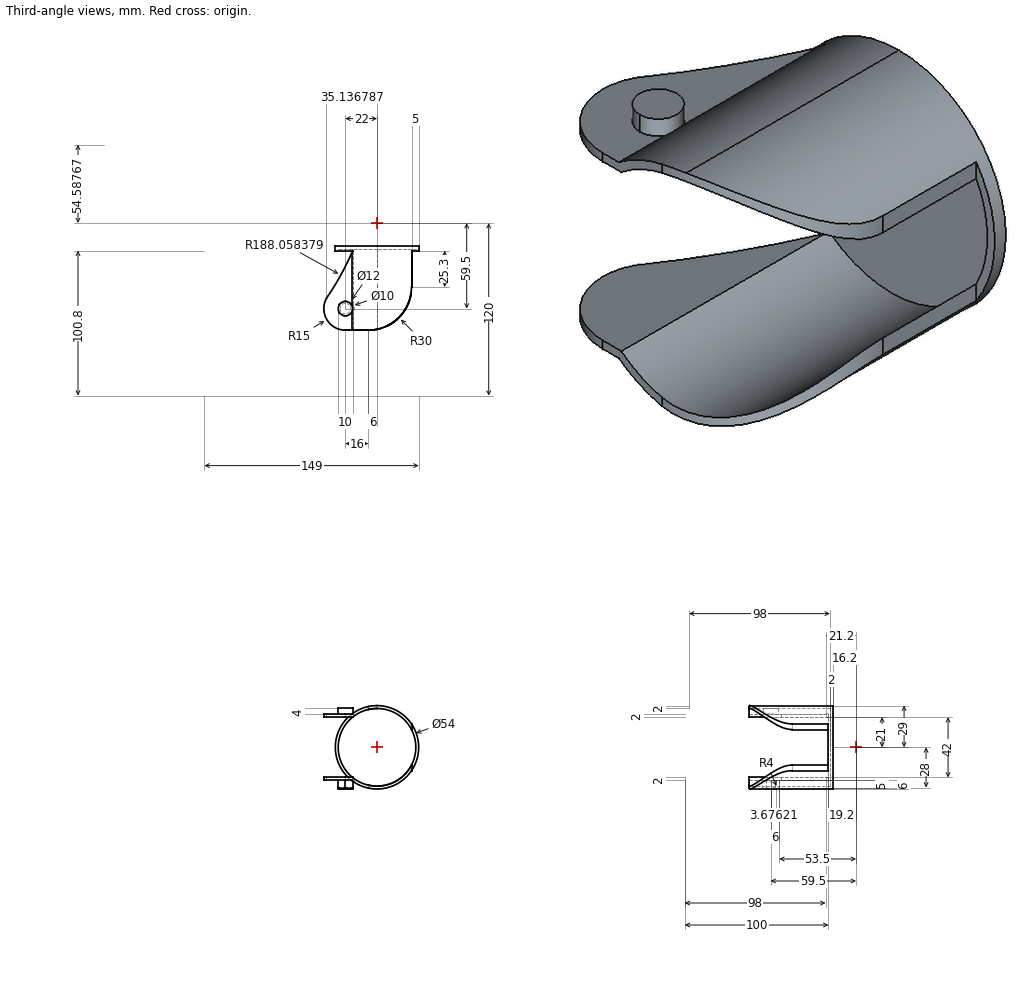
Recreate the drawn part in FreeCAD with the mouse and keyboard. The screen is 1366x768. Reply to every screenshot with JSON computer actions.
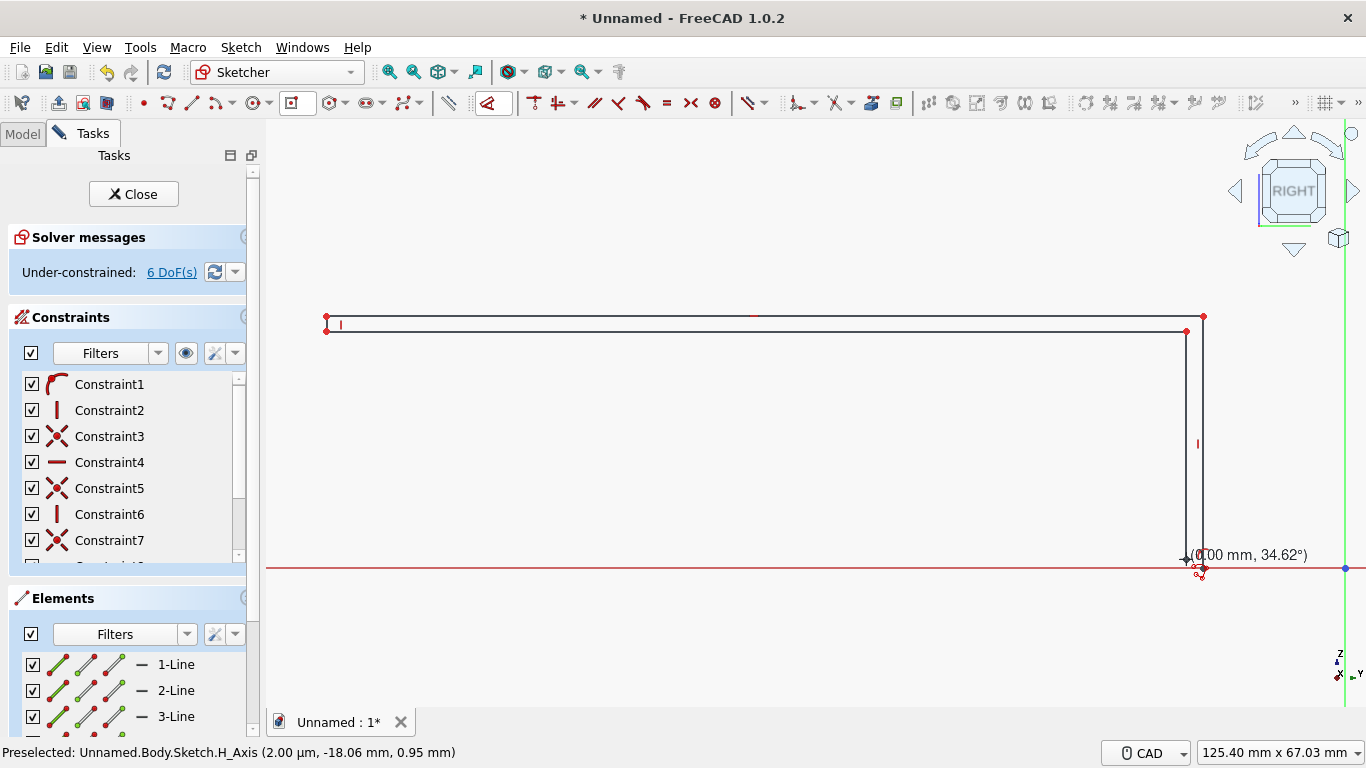
{"action": "scroll", "coordinate": [568, 356], "scroll_direction": "down", "scroll_amount": 2}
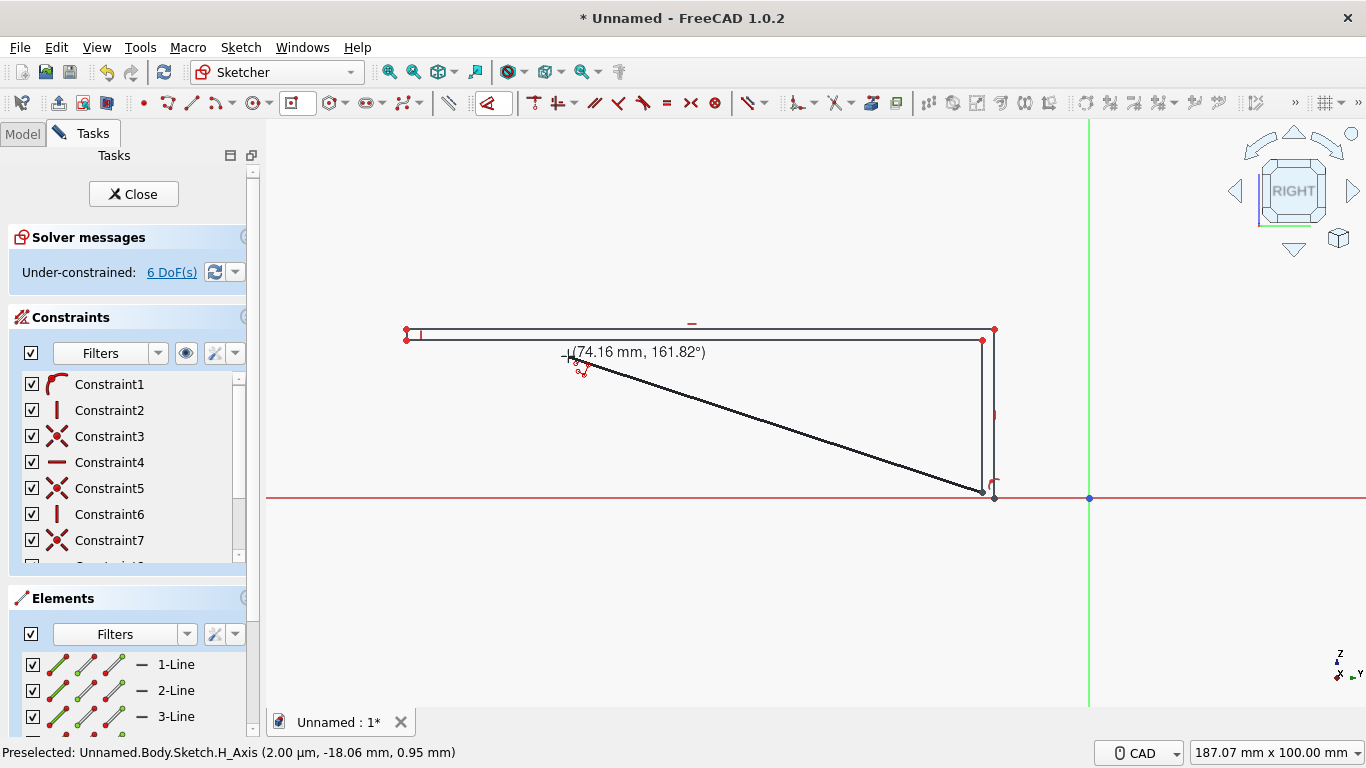
{"action": "scroll", "coordinate": [994, 498], "scroll_direction": "up", "scroll_amount": 2}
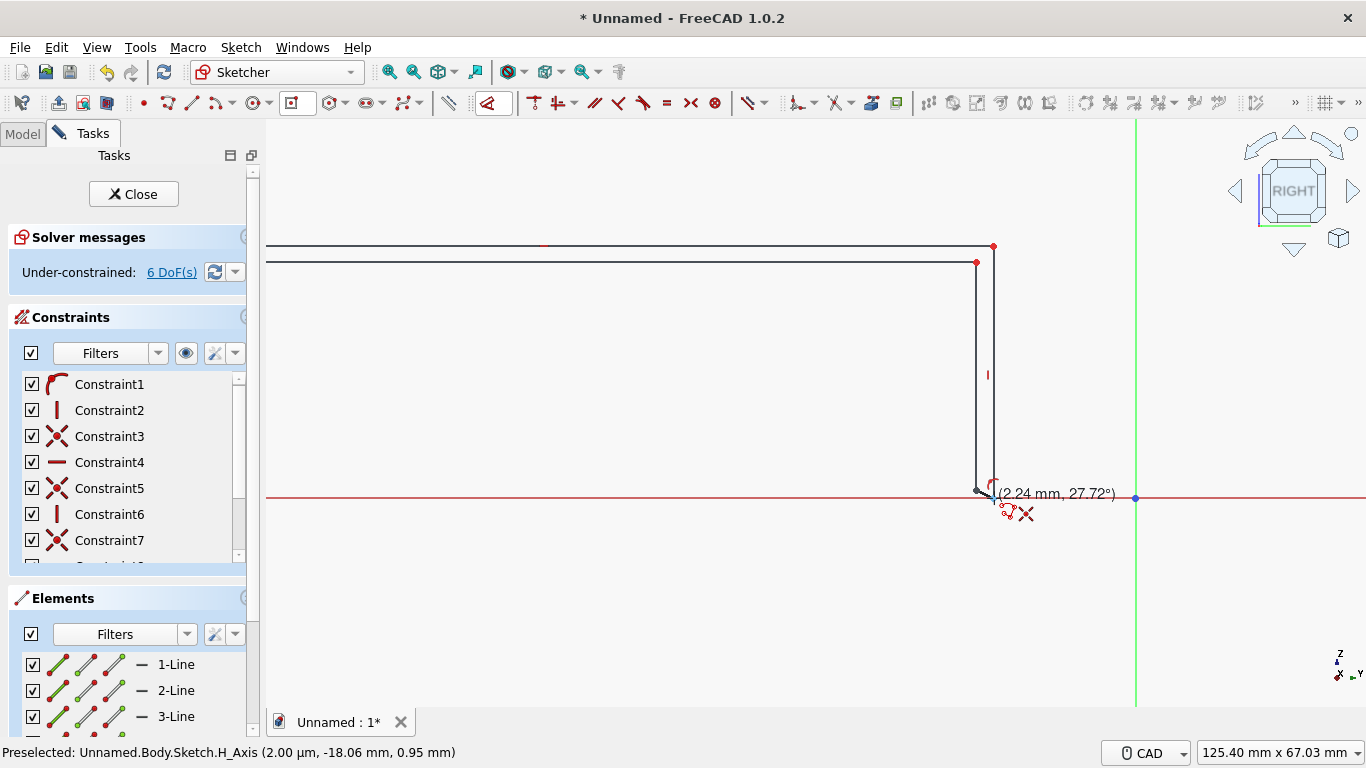
{"action": "left_click", "coordinate": [994, 498]}
{"action": "key", "text": "Escape"}
{"action": "key", "text": "Escape"}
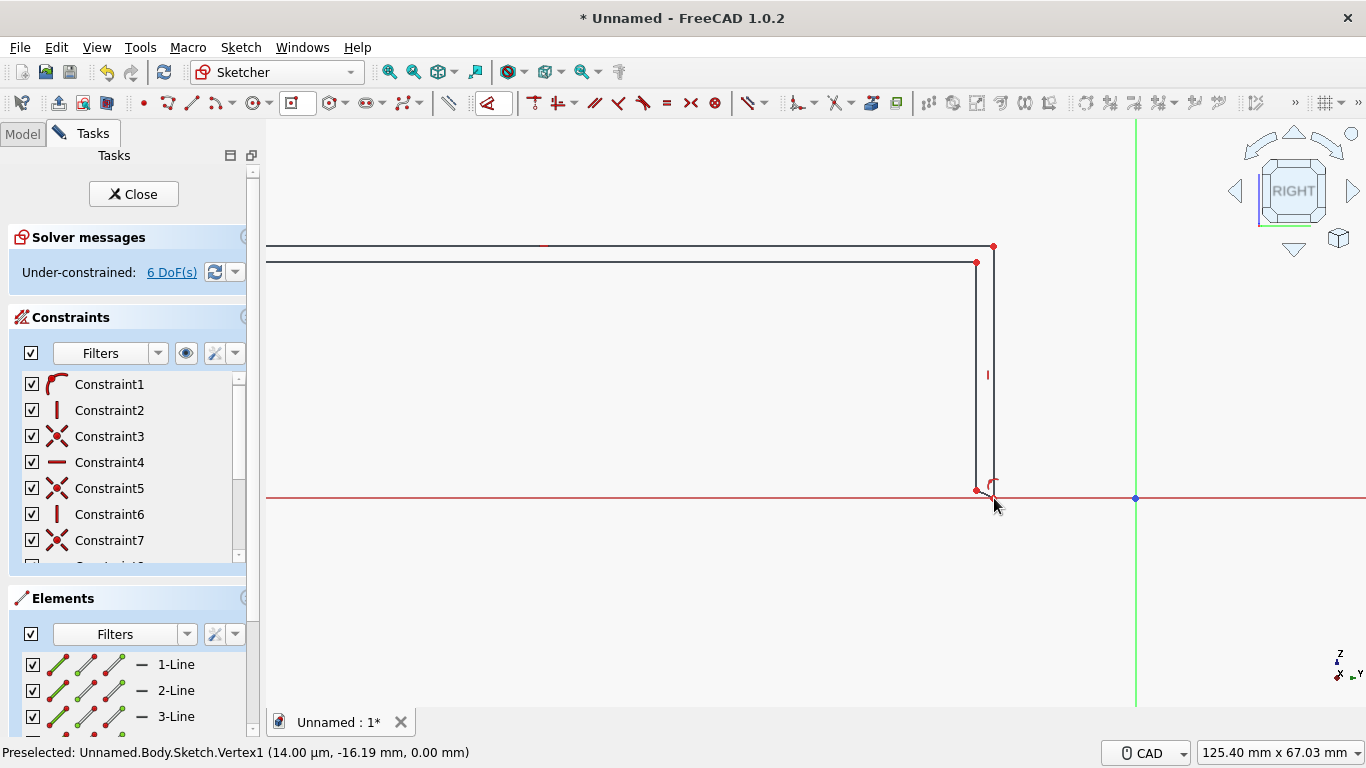
{"action": "scroll", "coordinate": [987, 495], "scroll_direction": "up", "scroll_amount": 4}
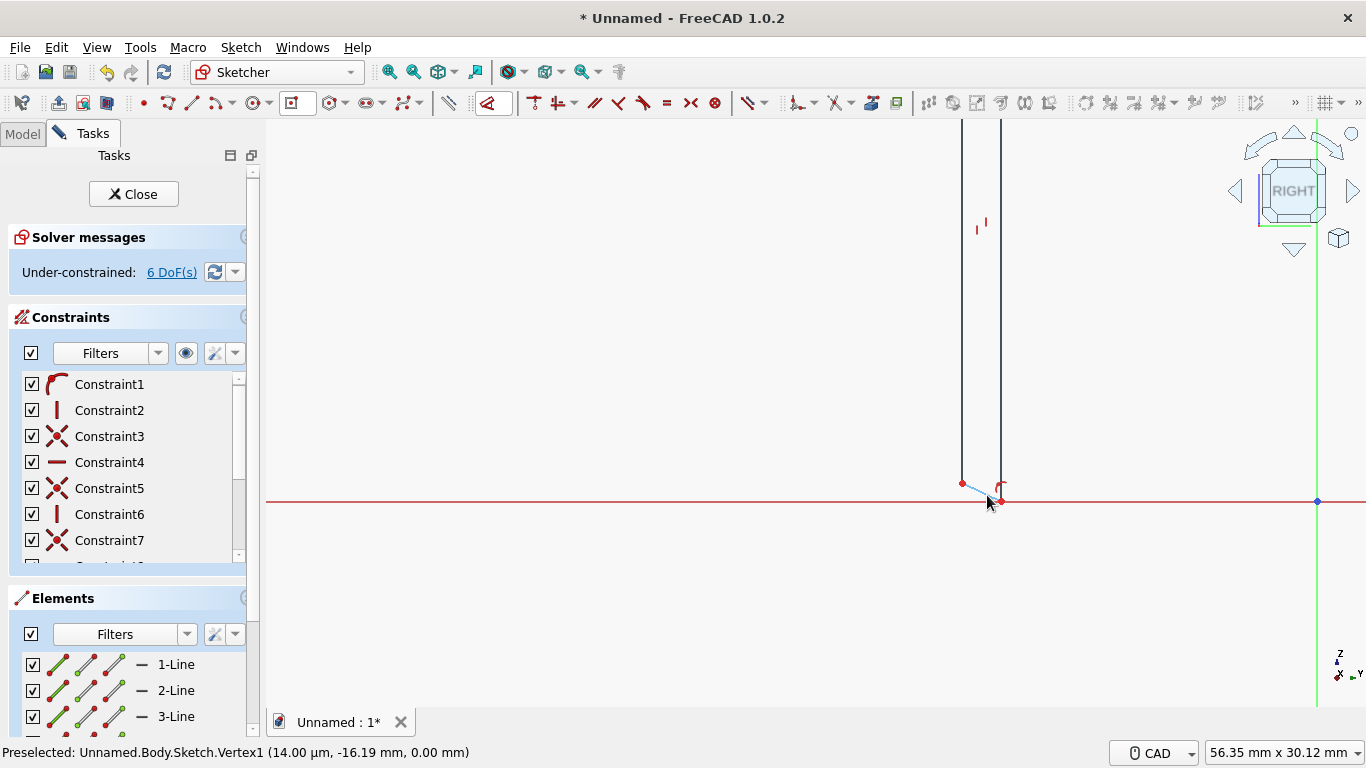
{"action": "left_click", "coordinate": [986, 494]}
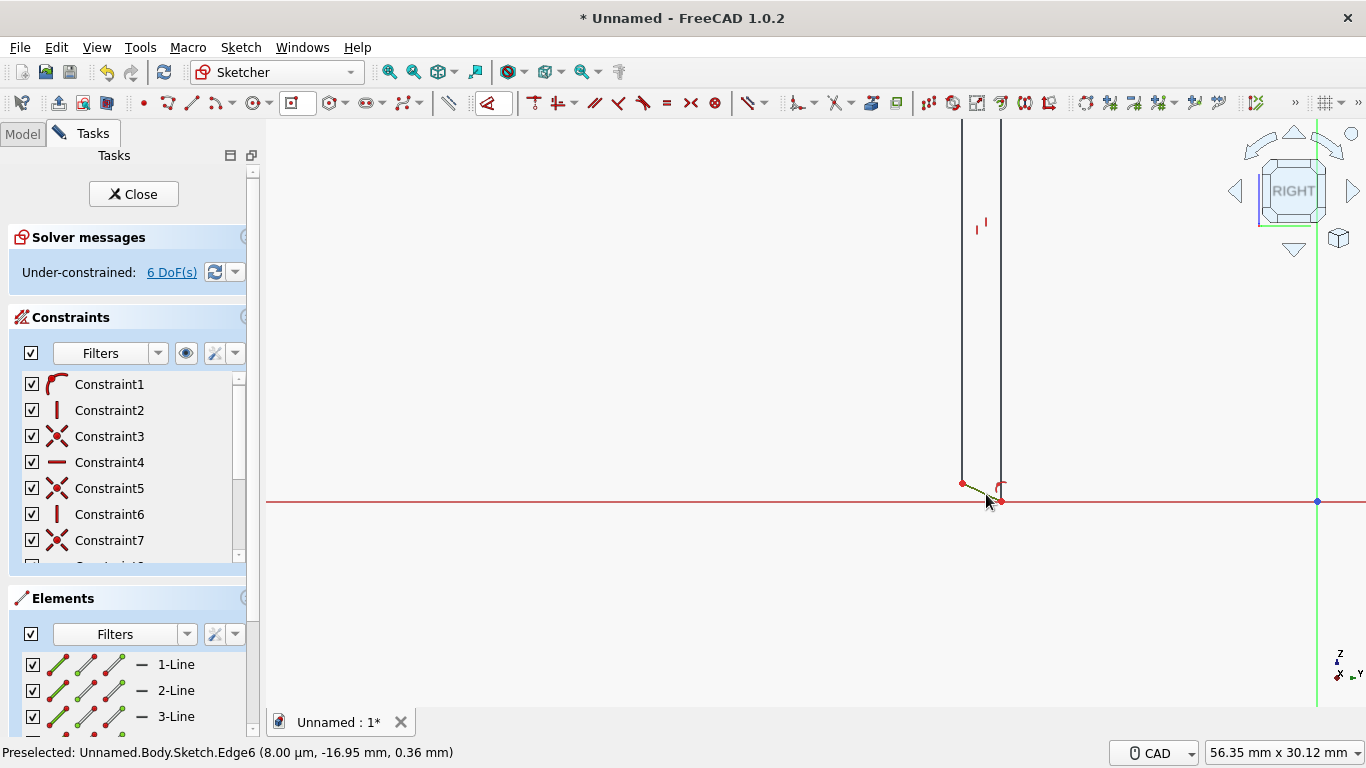
{"action": "key", "text": "h"}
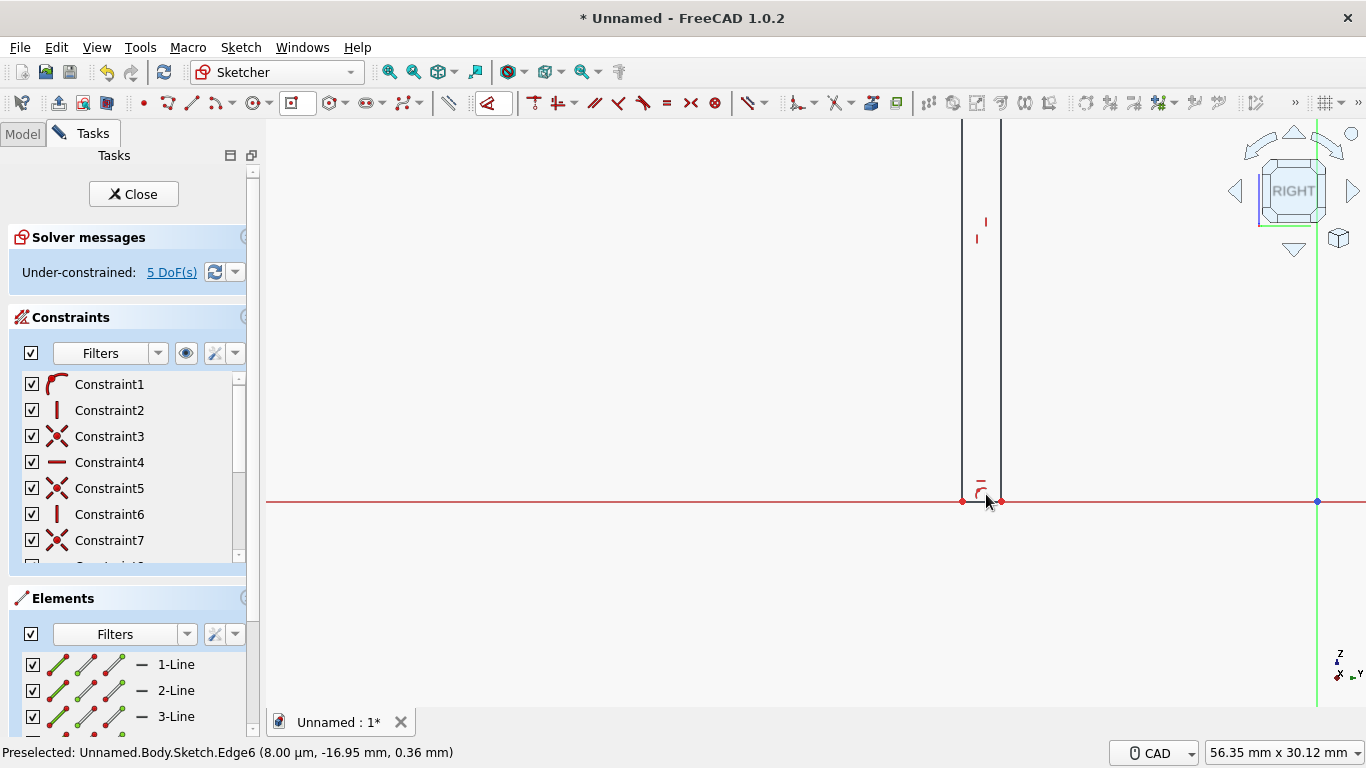
{"action": "left_click", "coordinate": [488, 104]}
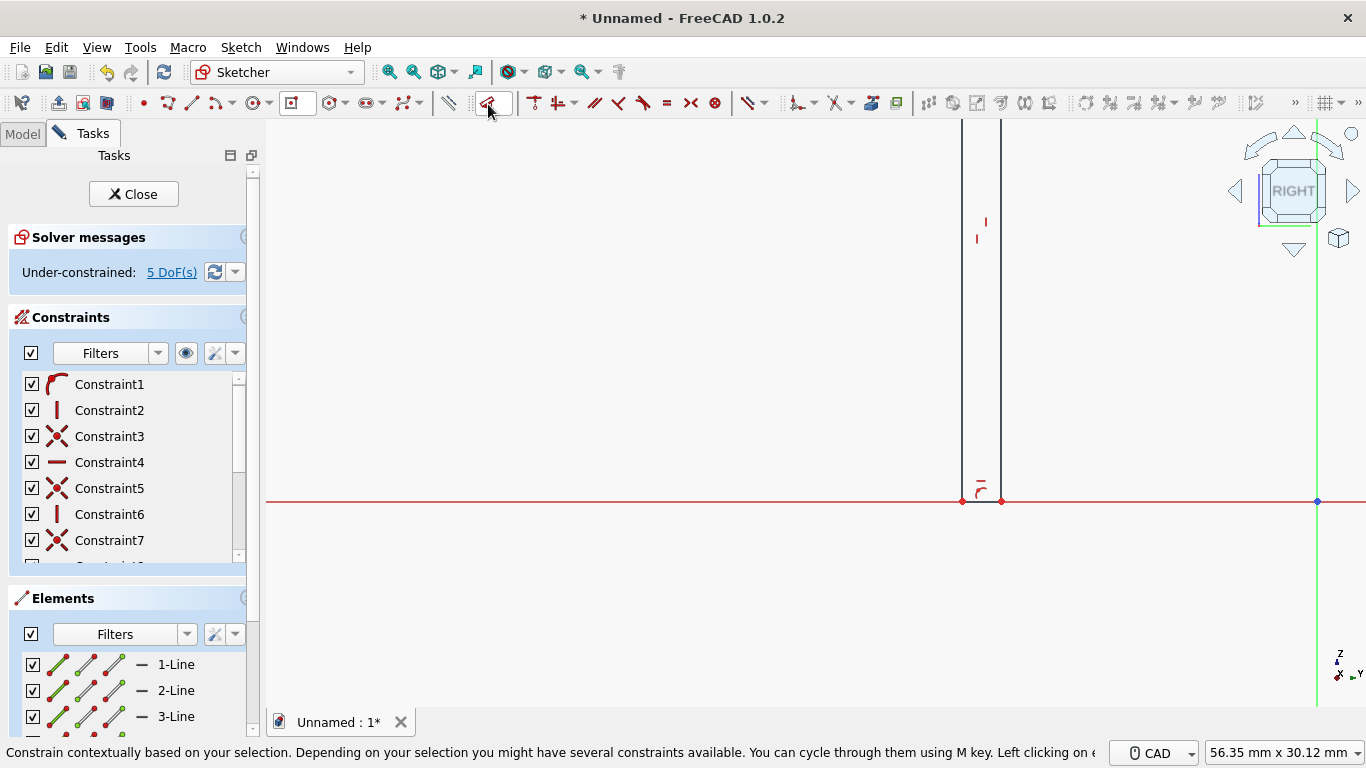
{"action": "scroll", "coordinate": [991, 497], "scroll_direction": "down", "scroll_amount": 6}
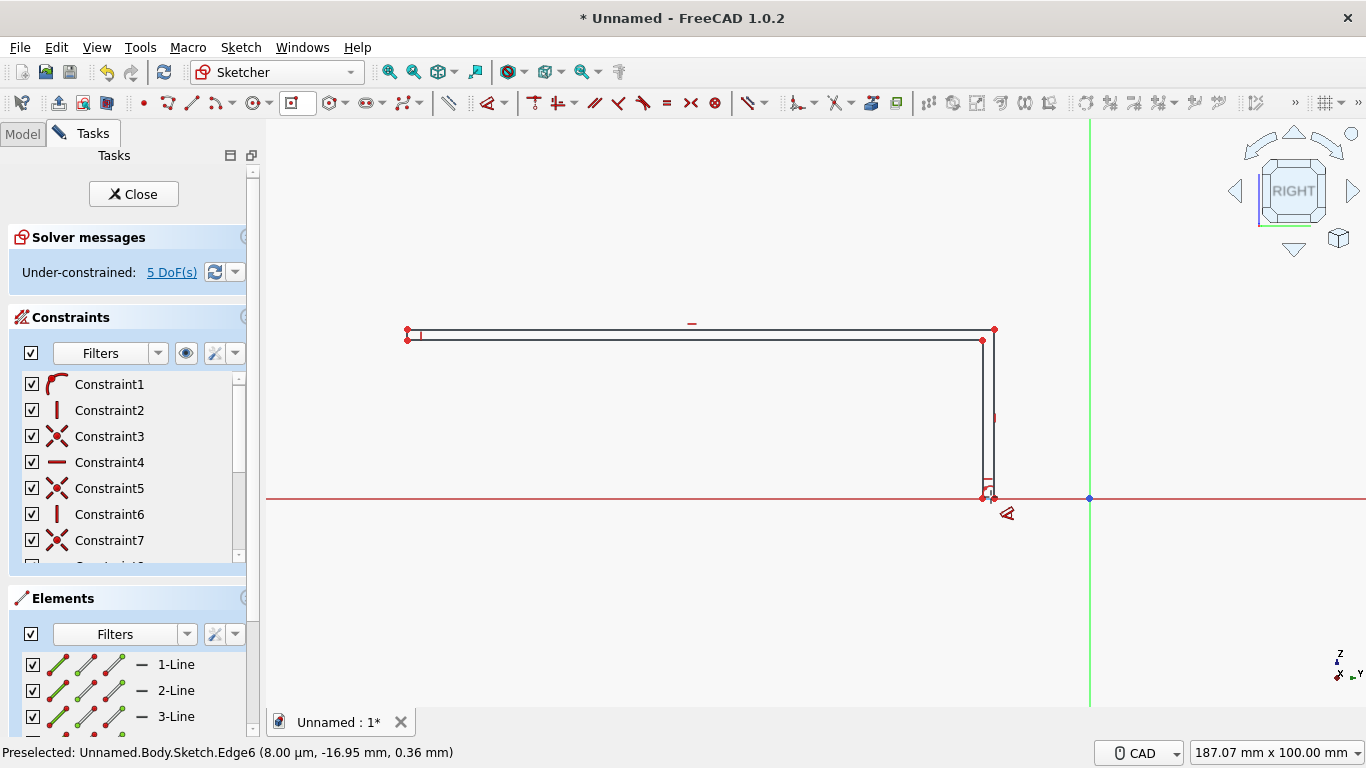
{"action": "scroll", "coordinate": [407, 333], "scroll_direction": "up", "scroll_amount": 8}